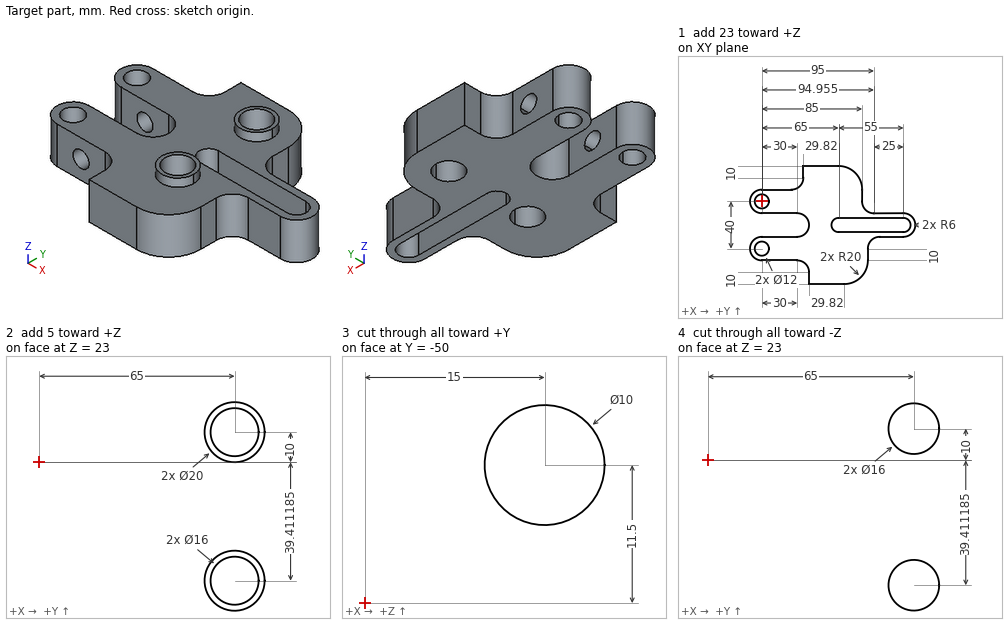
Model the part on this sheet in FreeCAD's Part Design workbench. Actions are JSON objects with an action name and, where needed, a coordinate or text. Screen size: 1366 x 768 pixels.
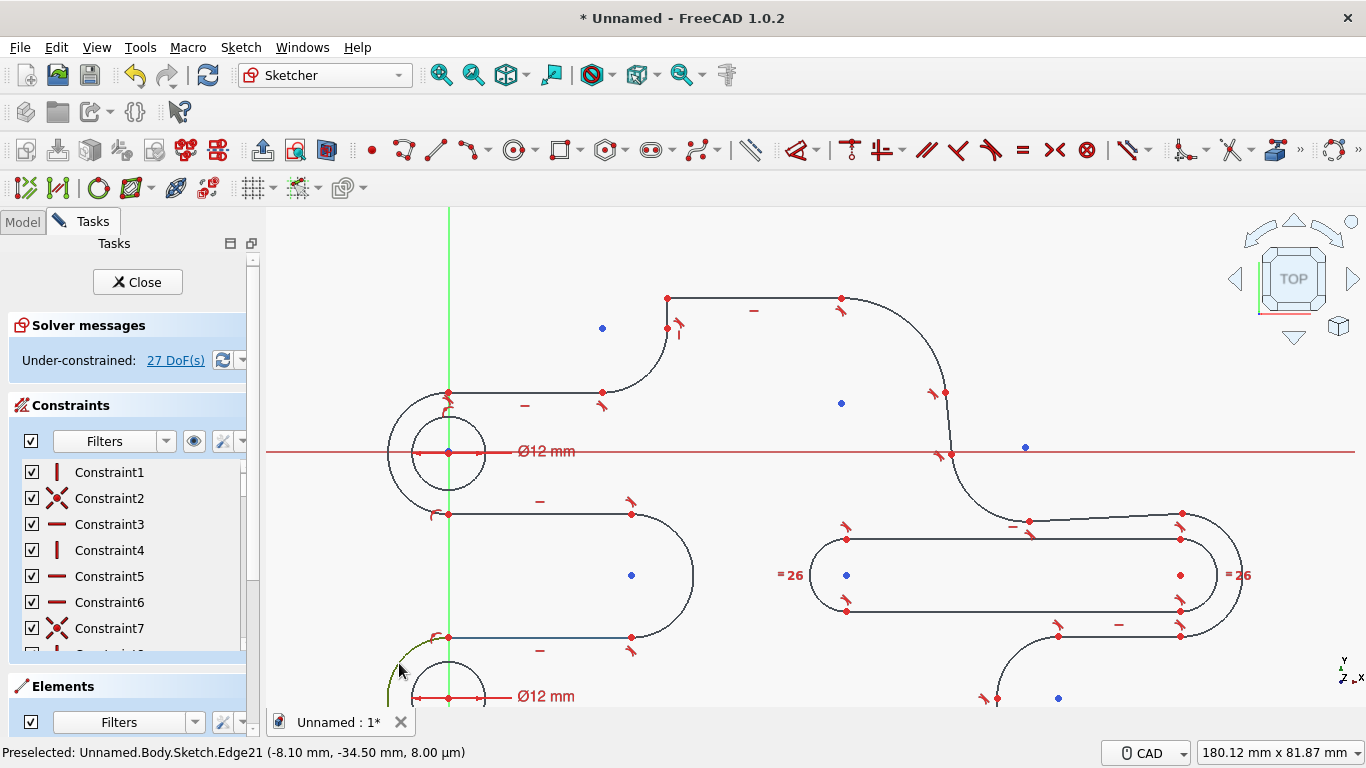
{"action": "key", "text": "t"}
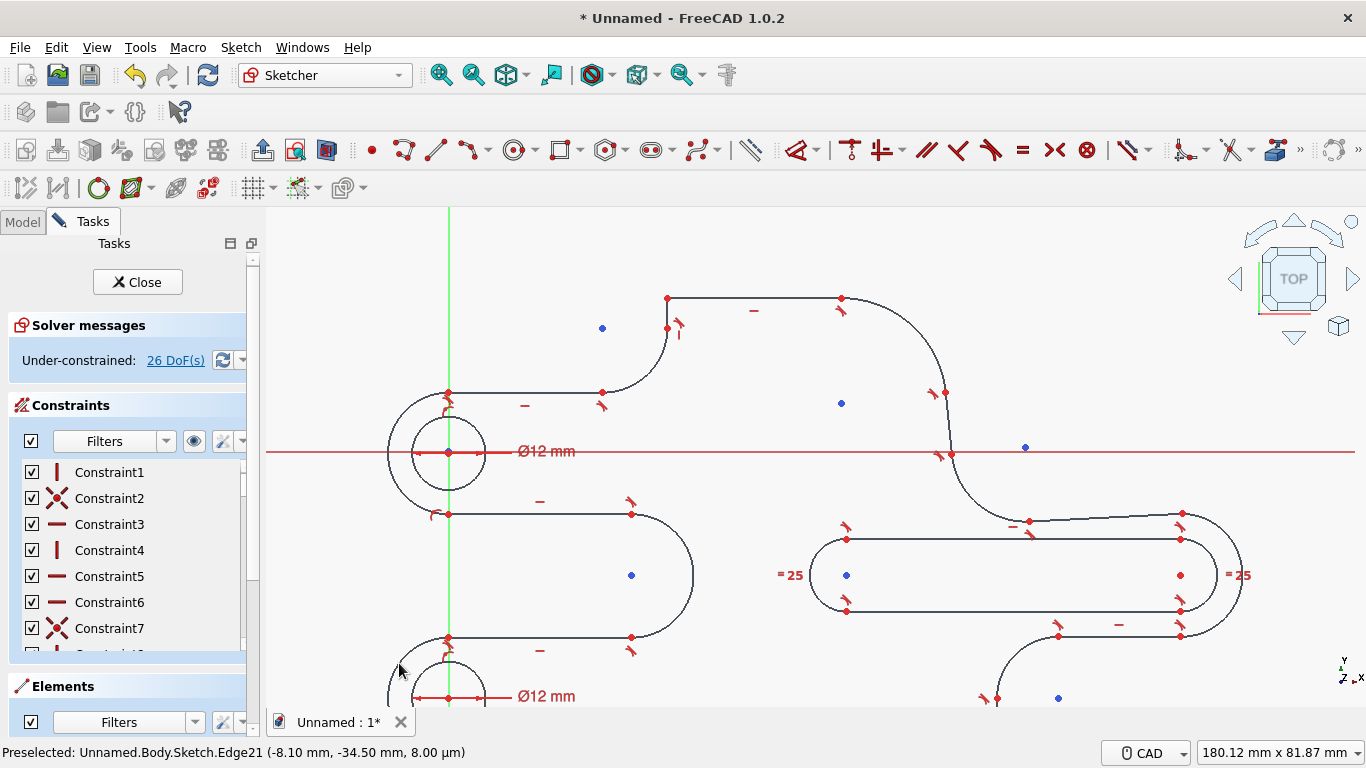
{"action": "scroll", "coordinate": [665, 315], "scroll_direction": "down", "scroll_amount": 3}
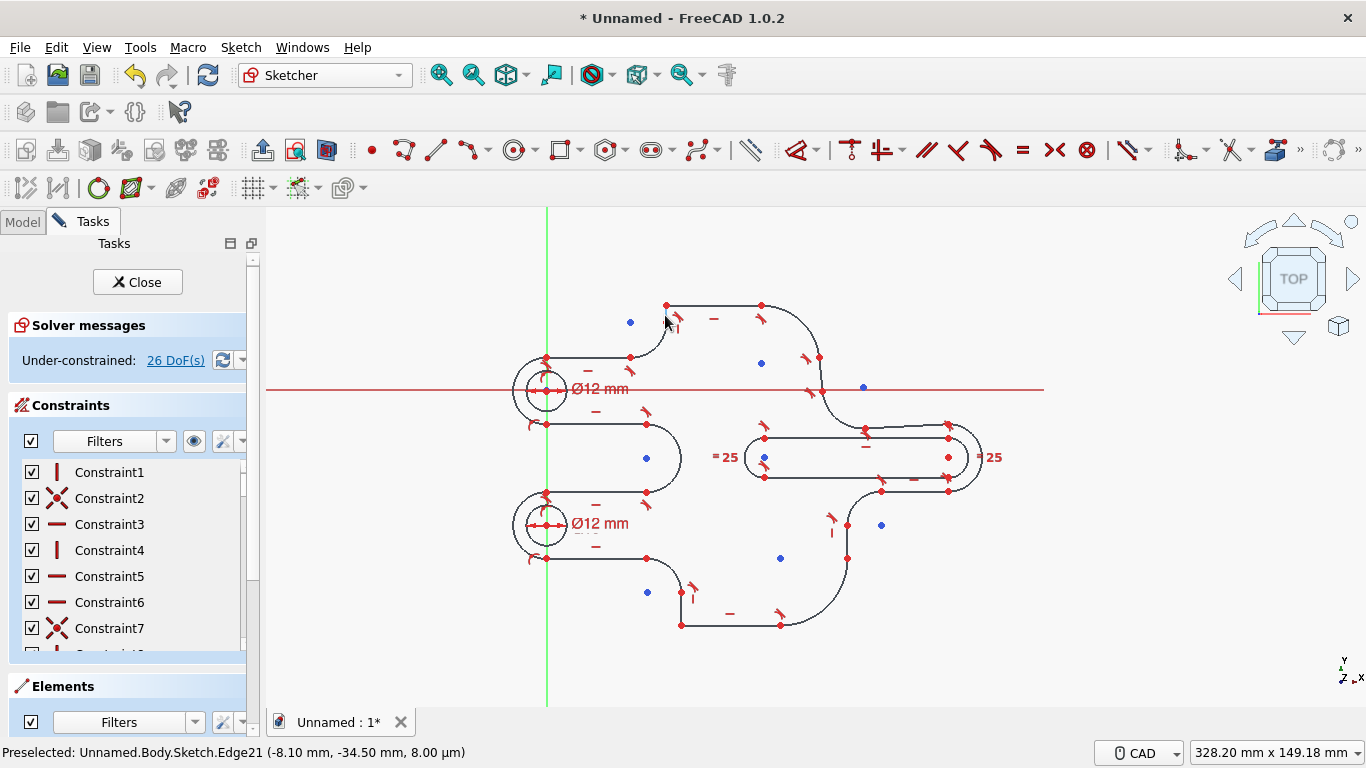
{"action": "left_click", "coordinate": [577, 559]}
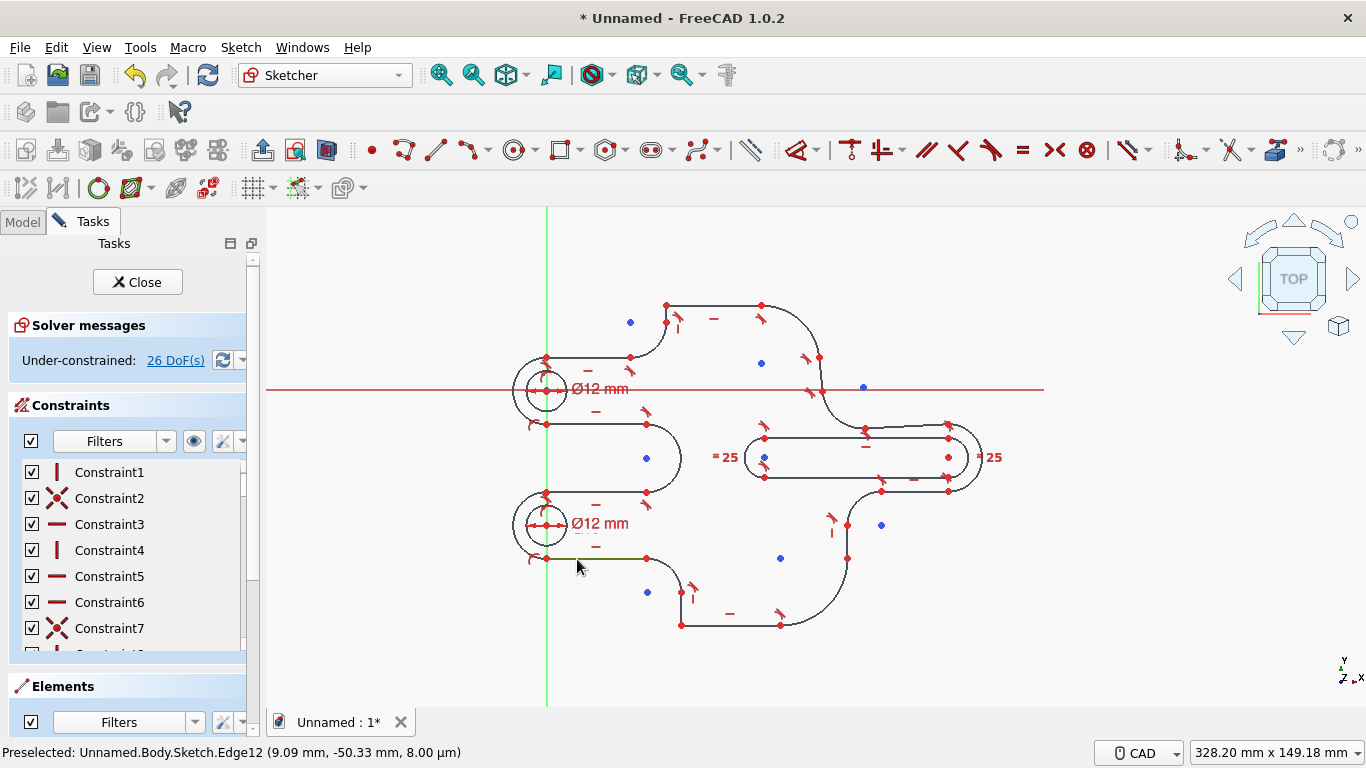
{"action": "left_click", "coordinate": [677, 577]}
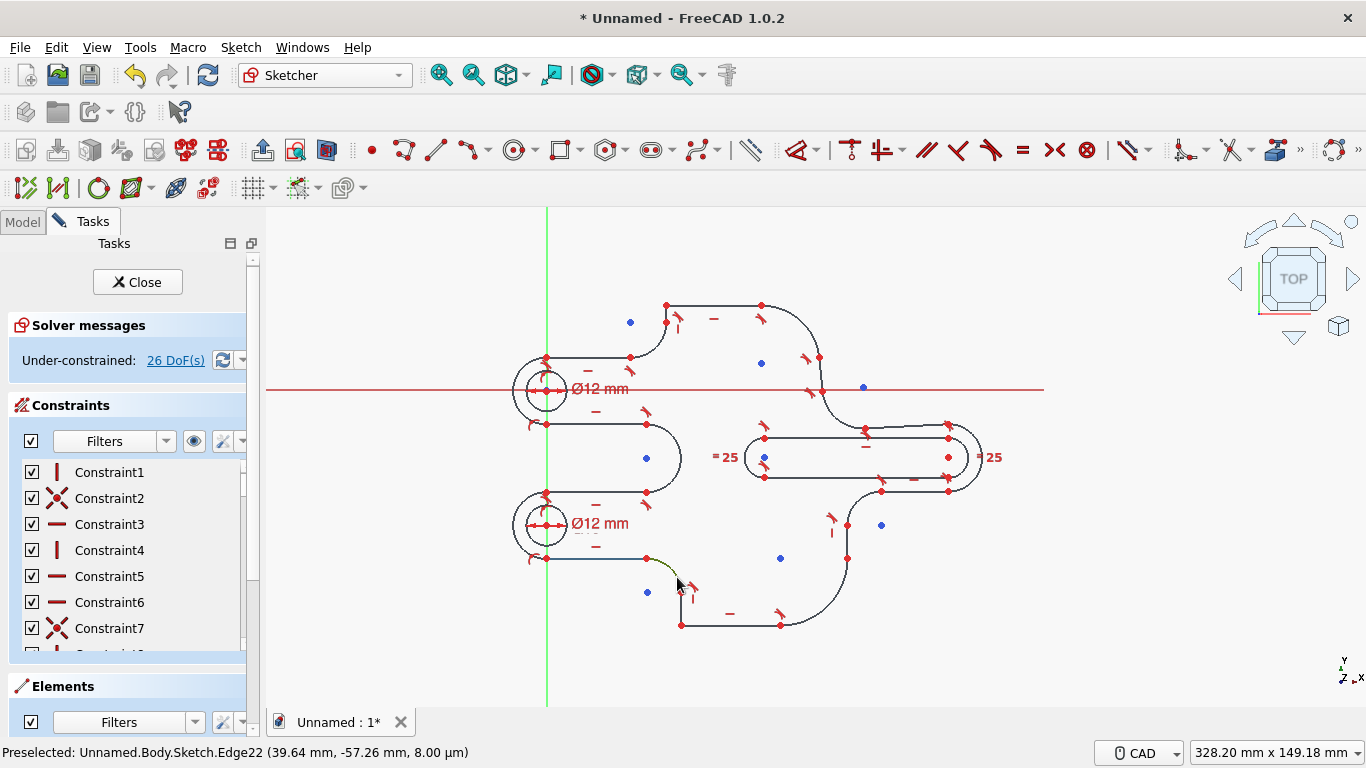
{"action": "left_click", "coordinate": [992, 150]}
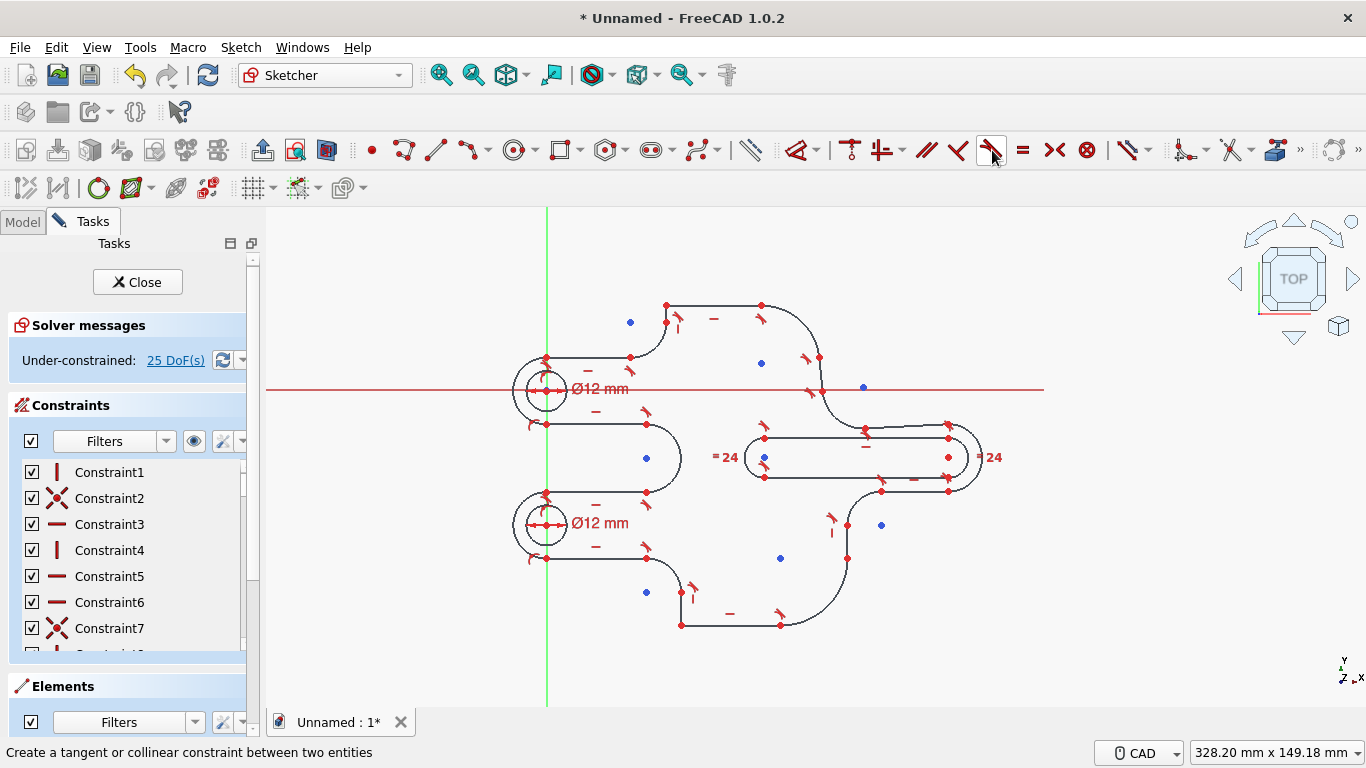
{"action": "left_click", "coordinate": [866, 495]}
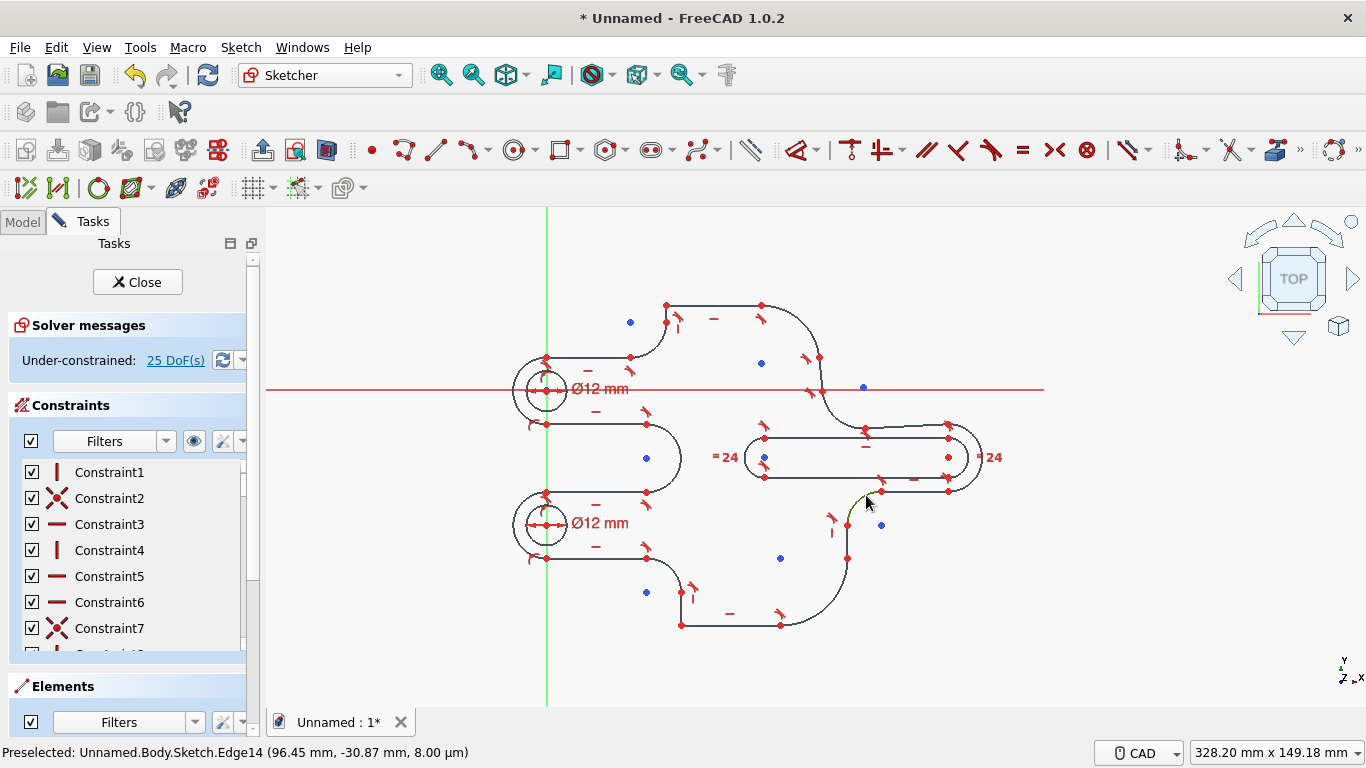
{"action": "left_click", "coordinate": [975, 478]}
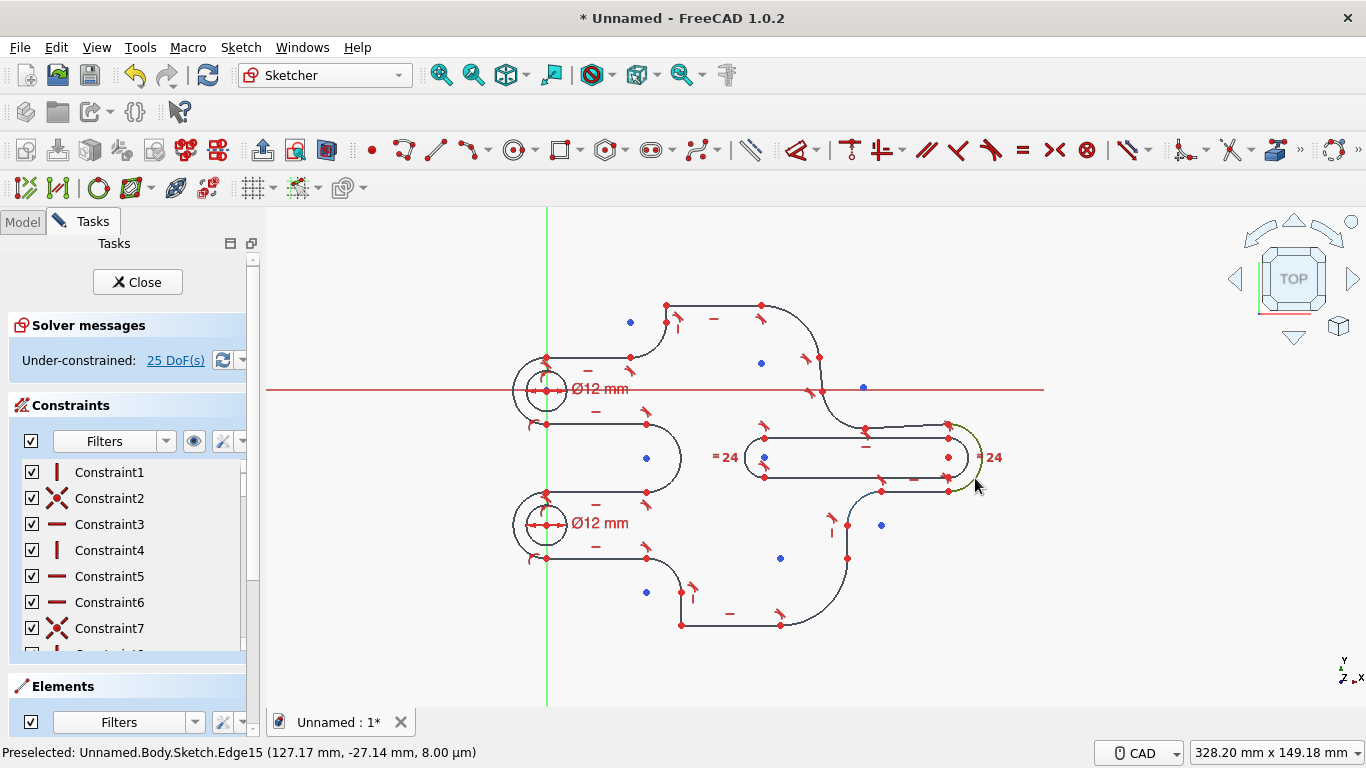
{"action": "left_click", "coordinate": [829, 409]}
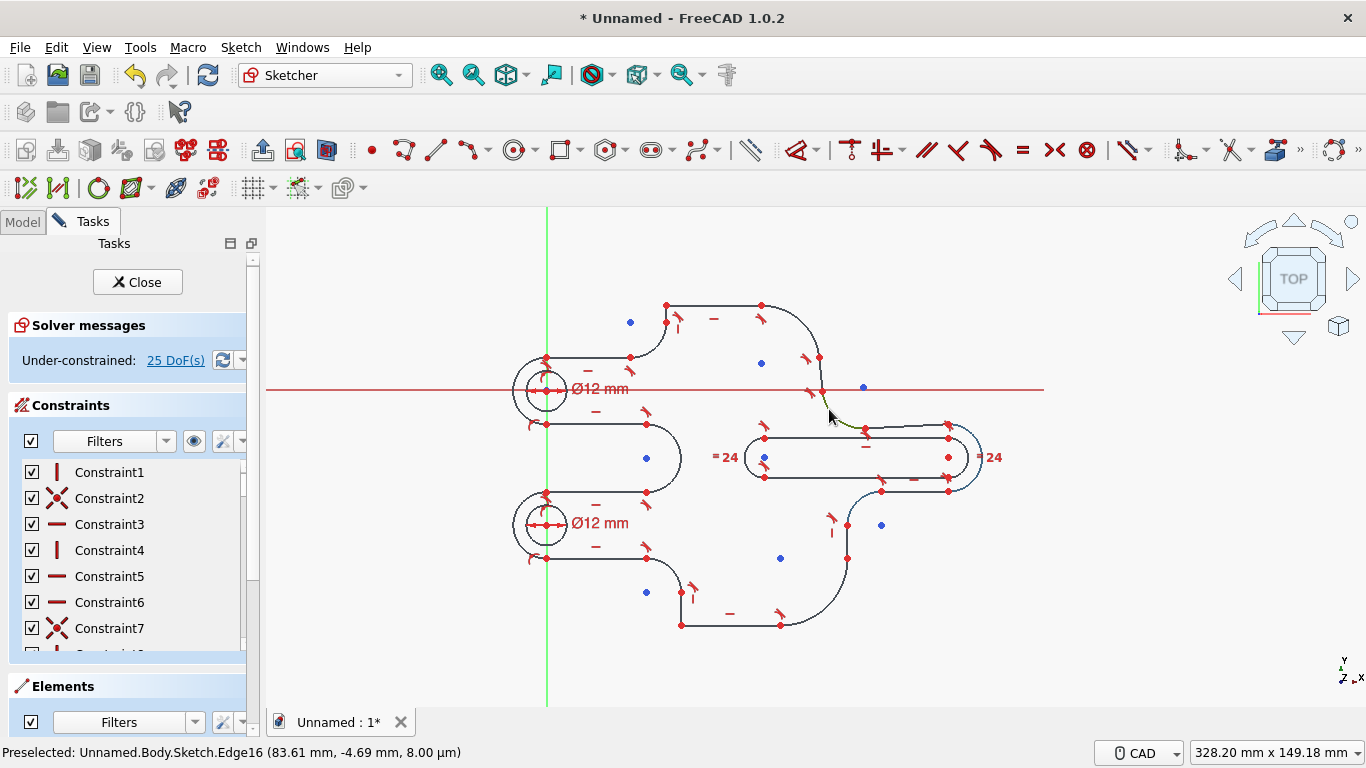
{"action": "left_click", "coordinate": [647, 354]}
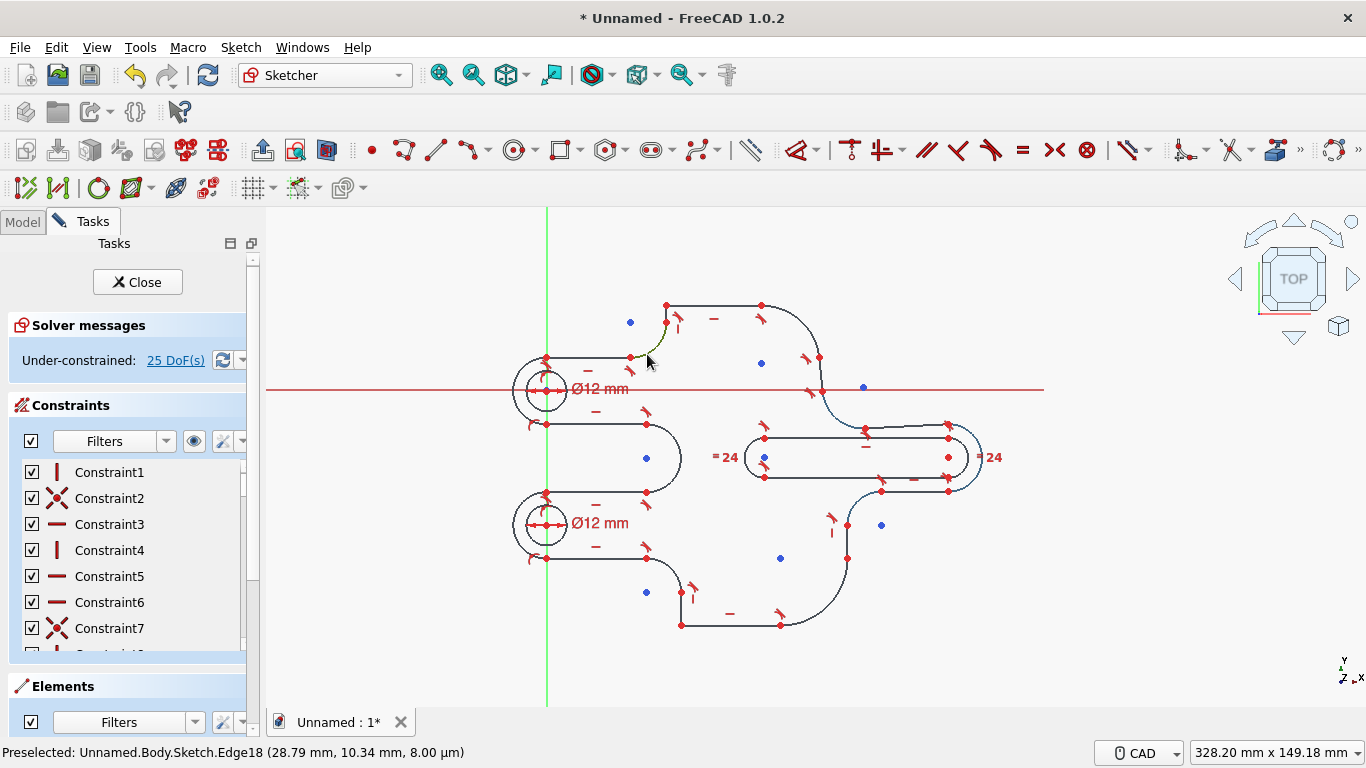
{"action": "left_click", "coordinate": [520, 371]}